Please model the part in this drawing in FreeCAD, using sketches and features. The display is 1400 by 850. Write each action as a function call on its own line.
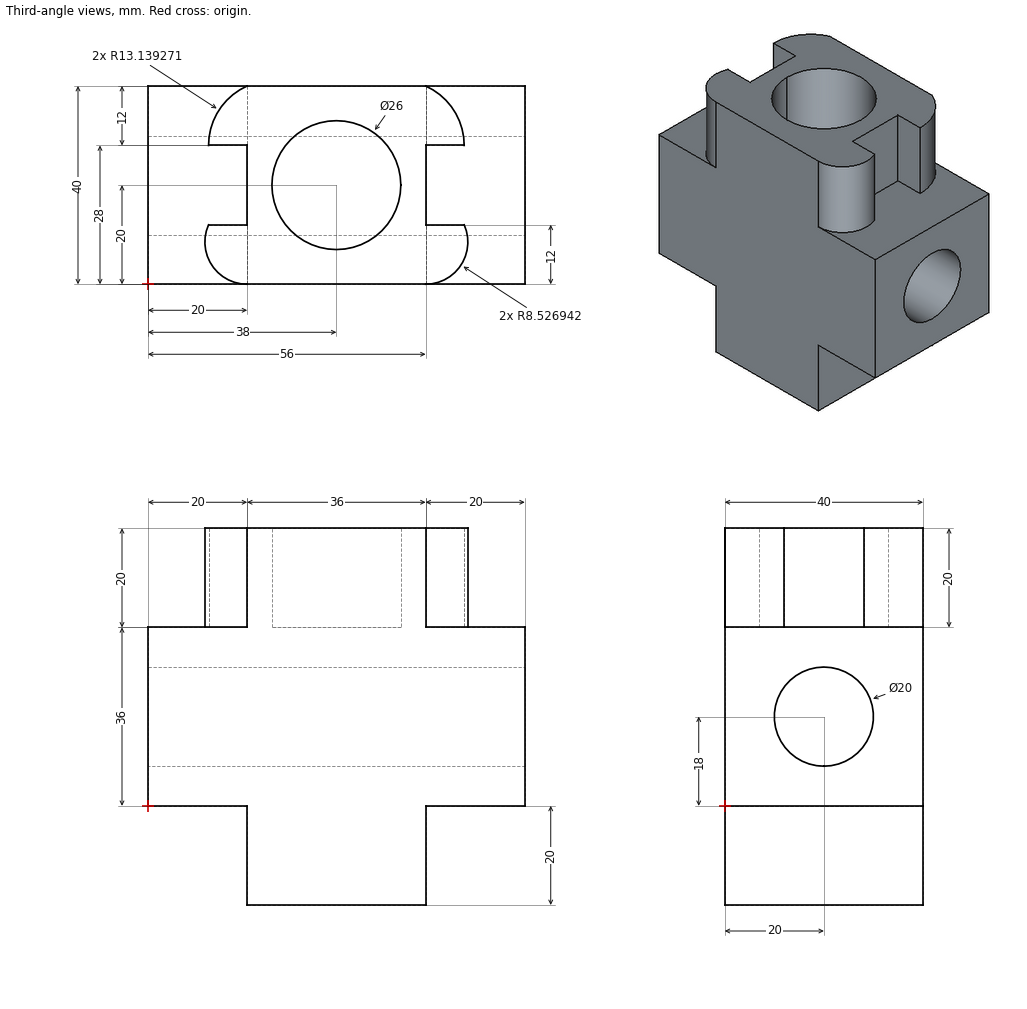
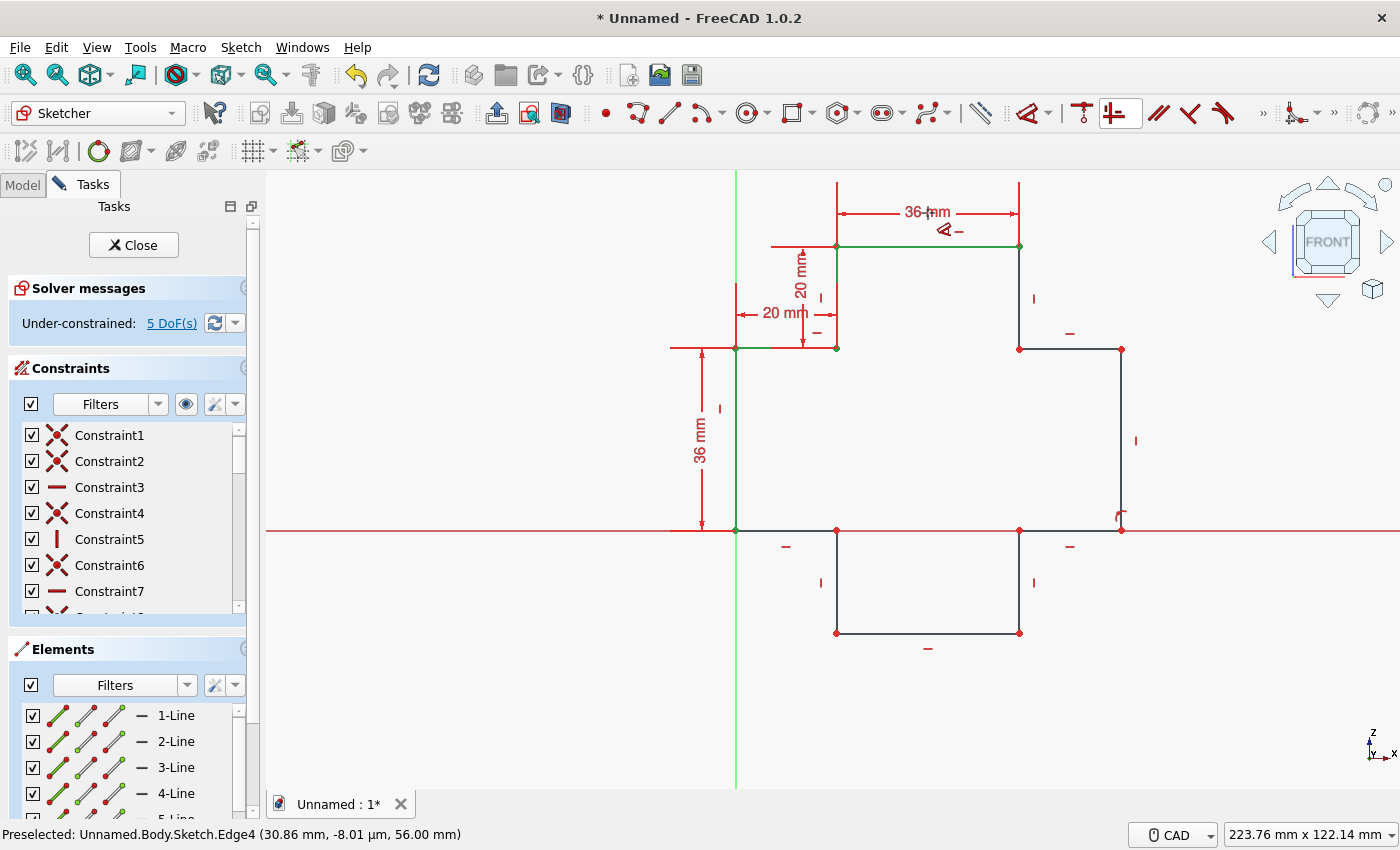
click(1019, 278)
click(1053, 298)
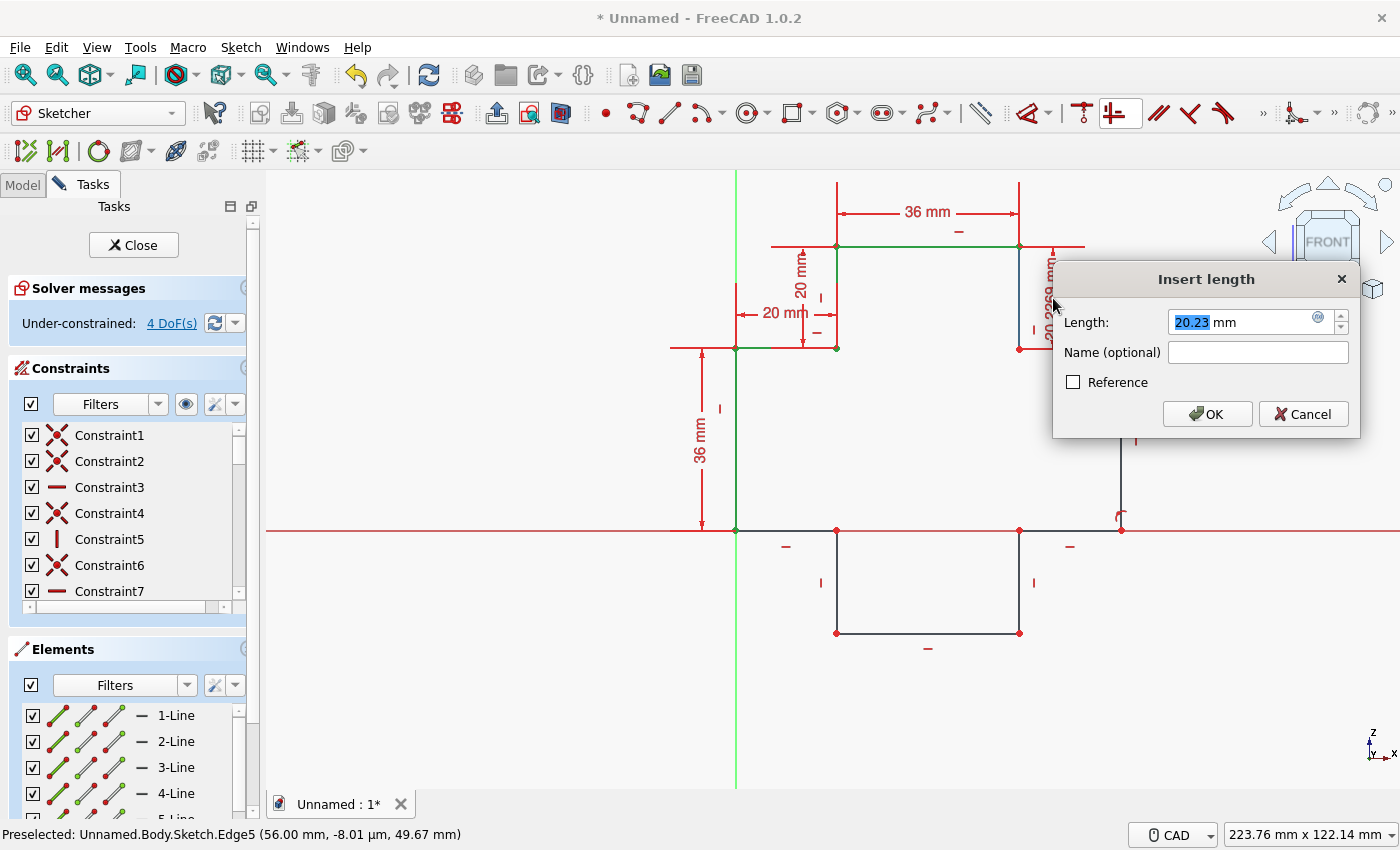
text(20)
key(Return)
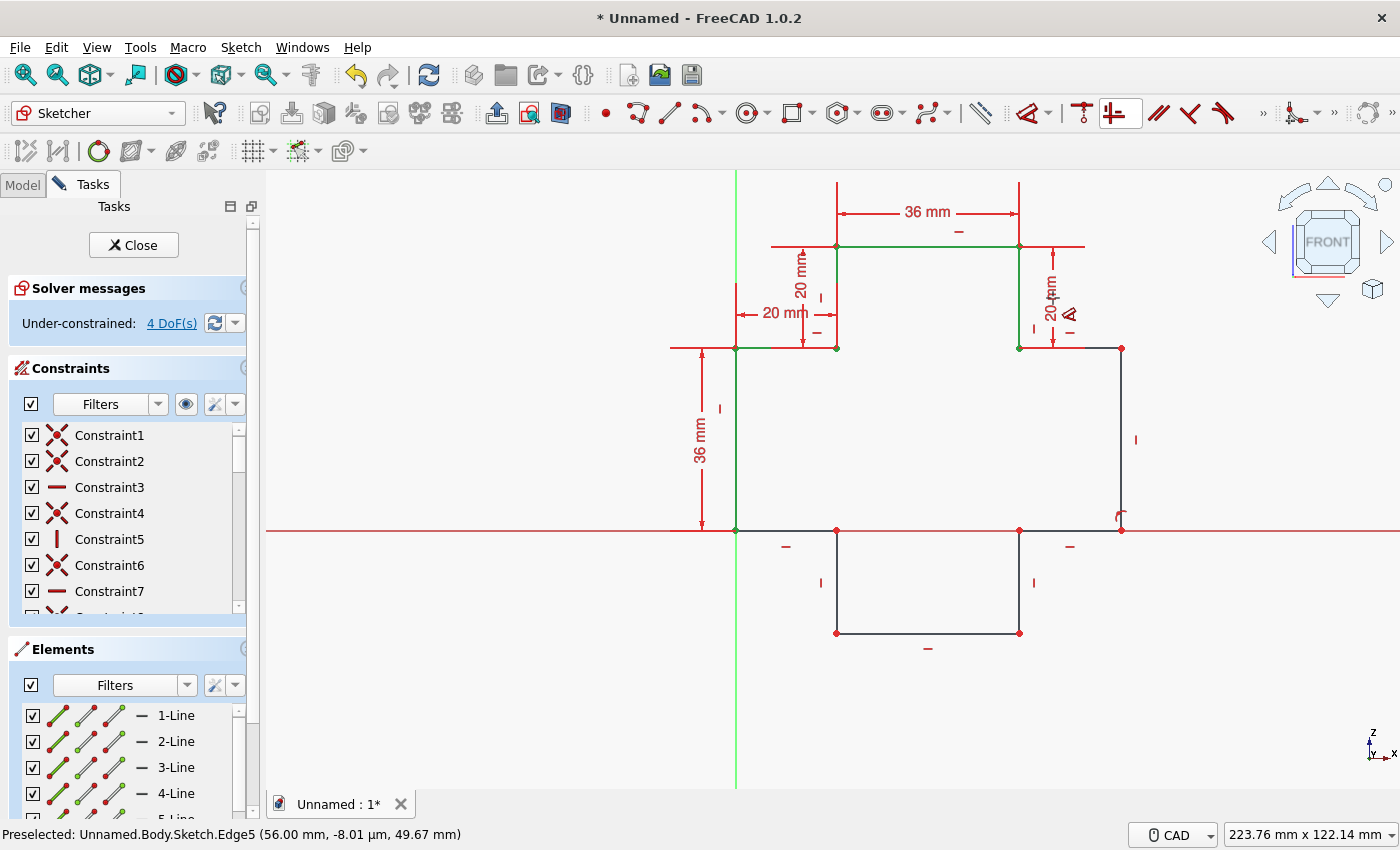
click(1050, 348)
click(1070, 382)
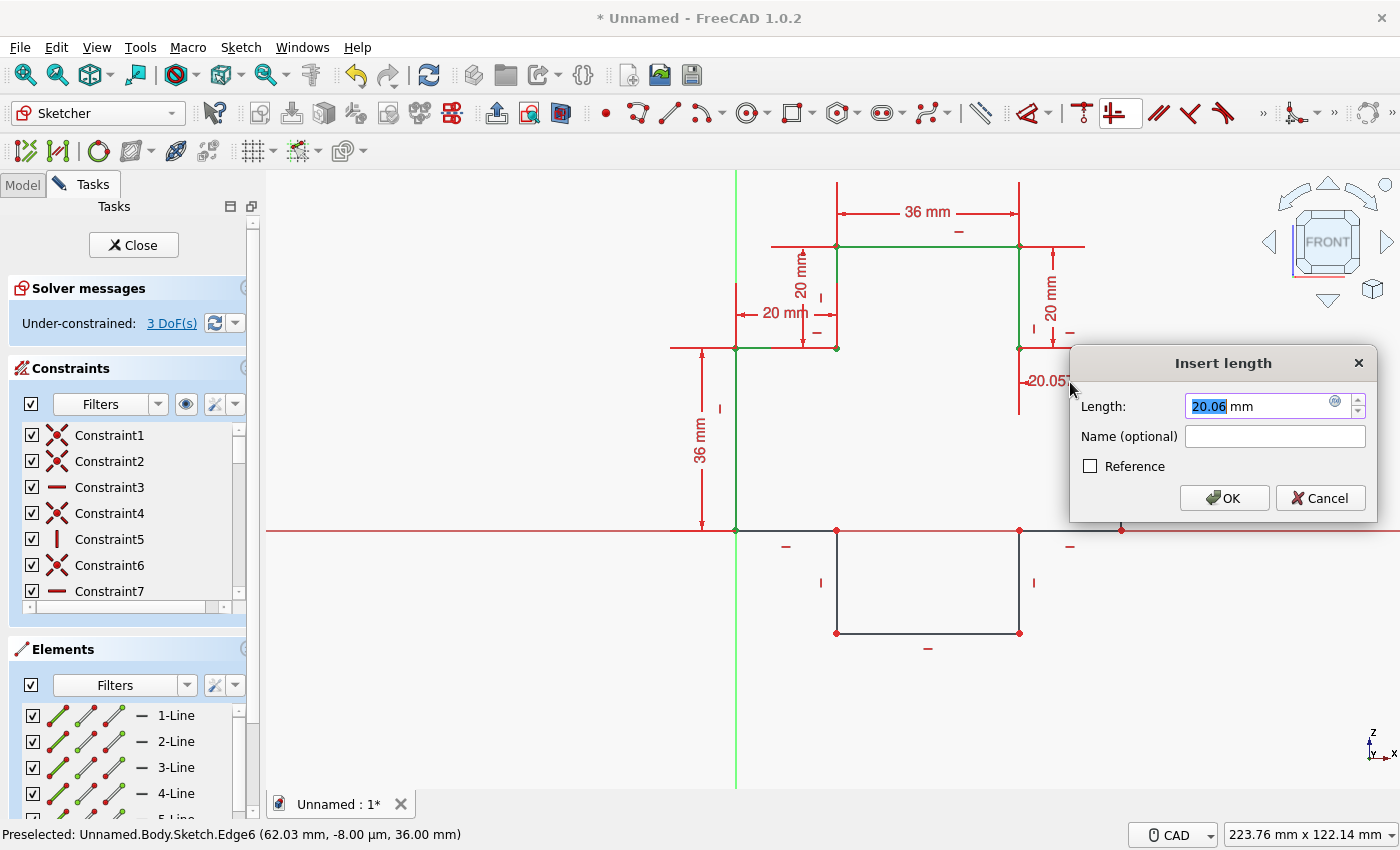
text(20)
key(Return)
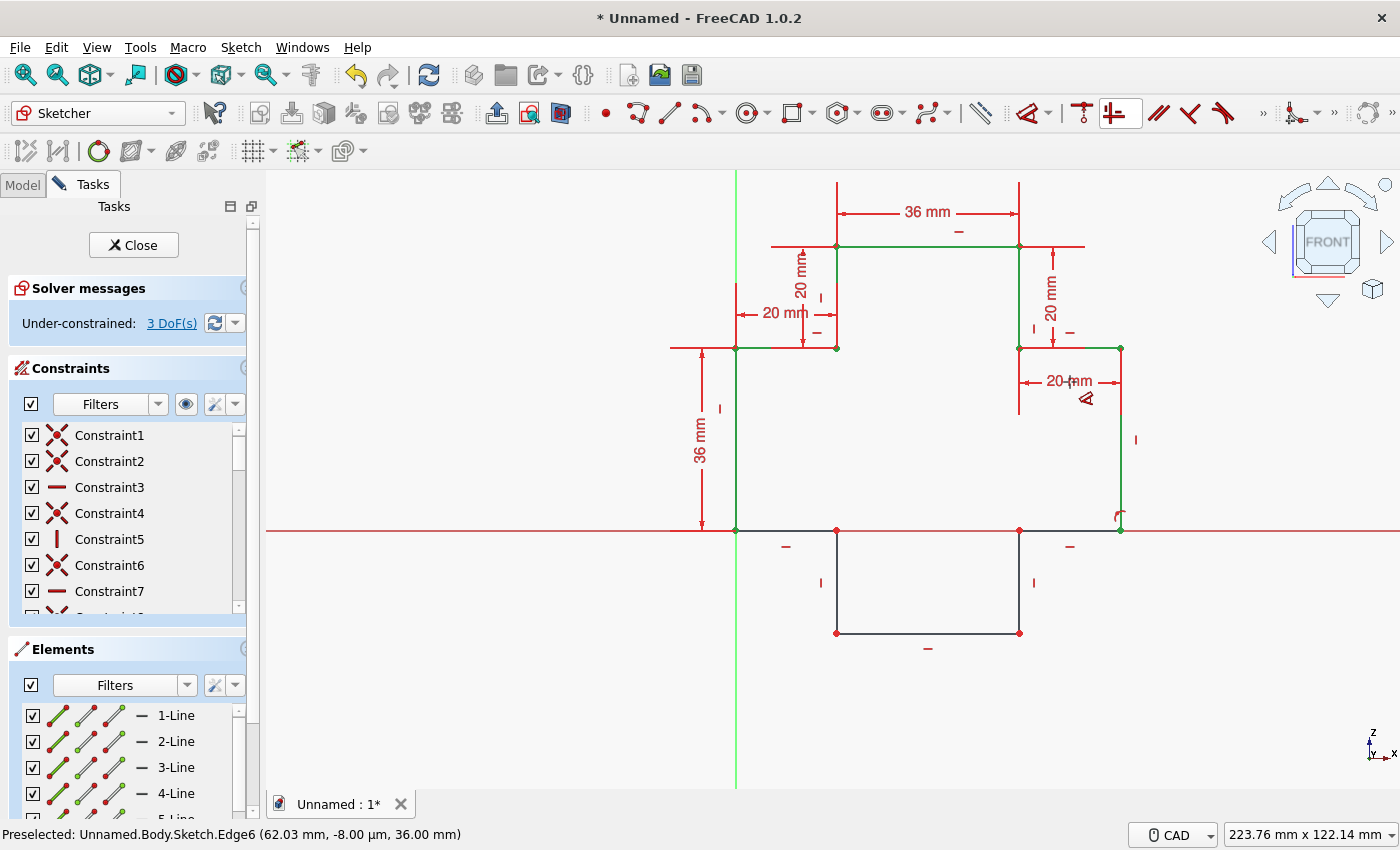
click(1090, 531)
click(1070, 565)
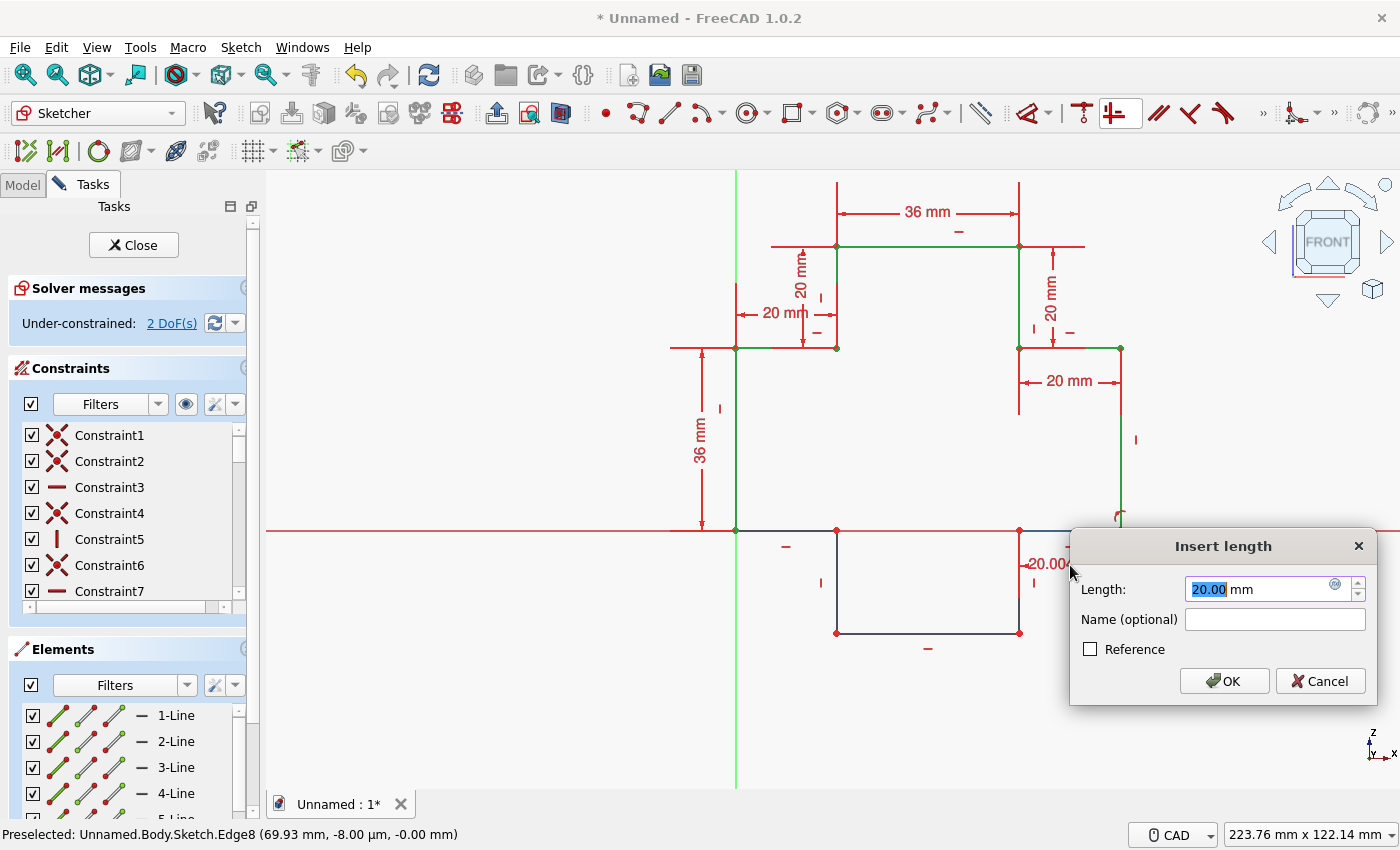
text(20)
key(Return)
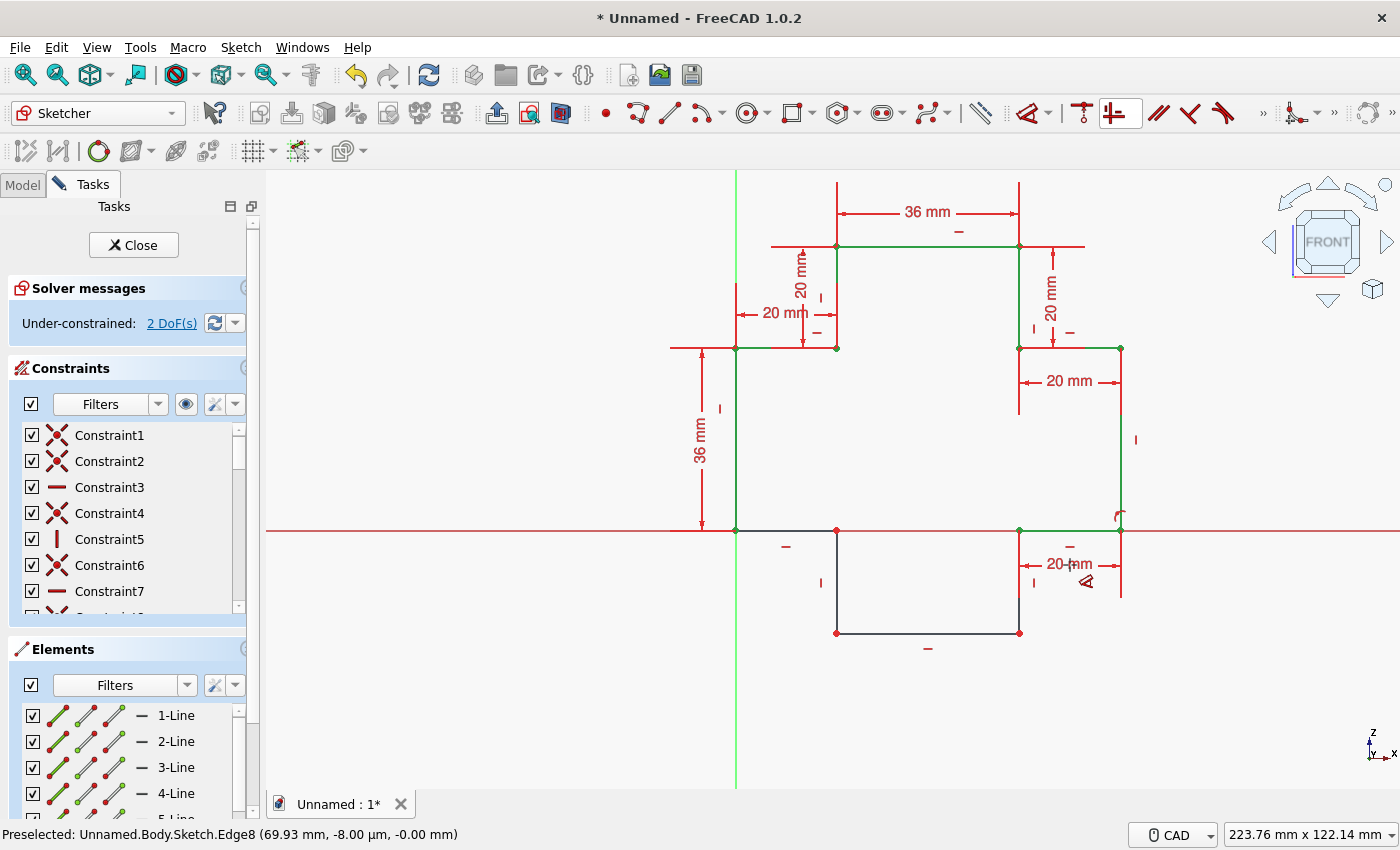
click(1019, 562)
click(1053, 606)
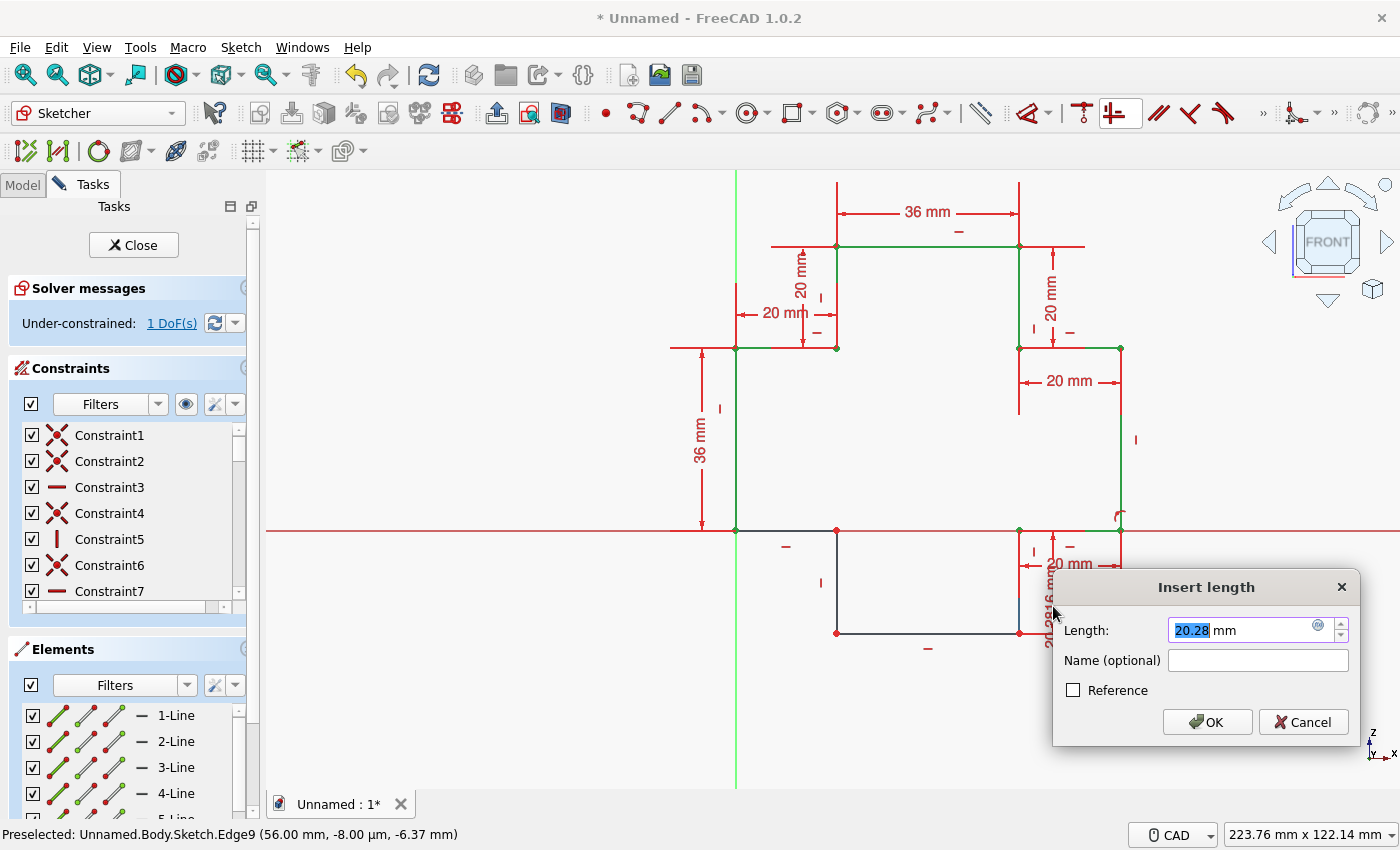
text(20)
key(Return)